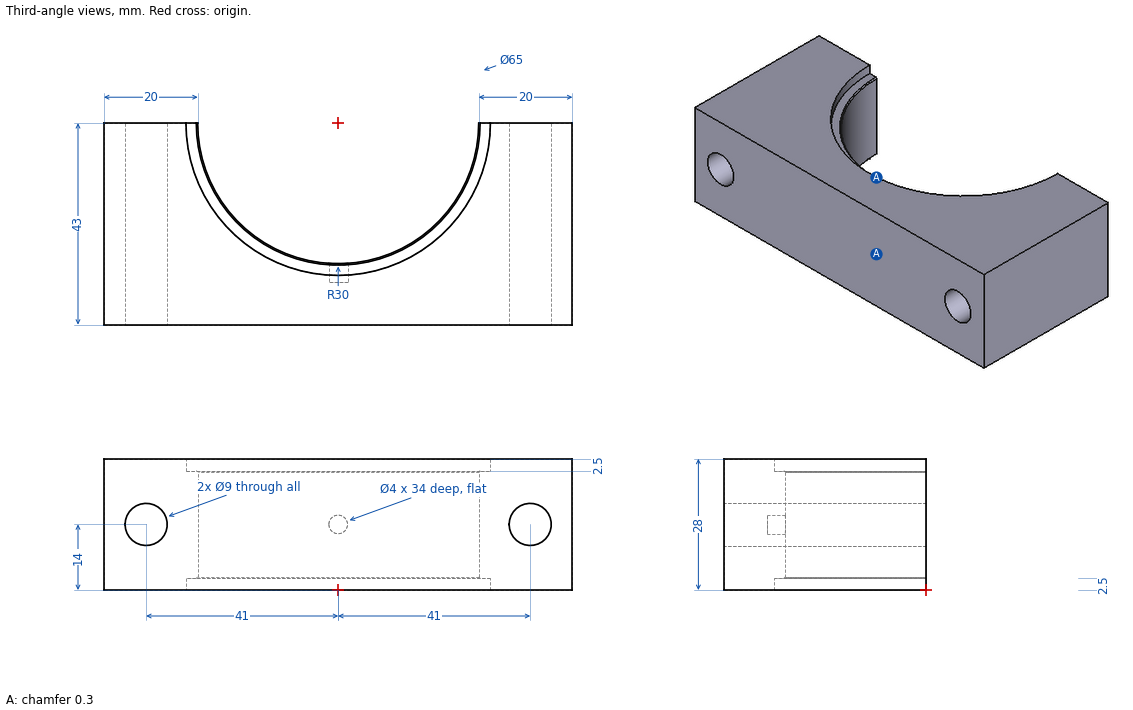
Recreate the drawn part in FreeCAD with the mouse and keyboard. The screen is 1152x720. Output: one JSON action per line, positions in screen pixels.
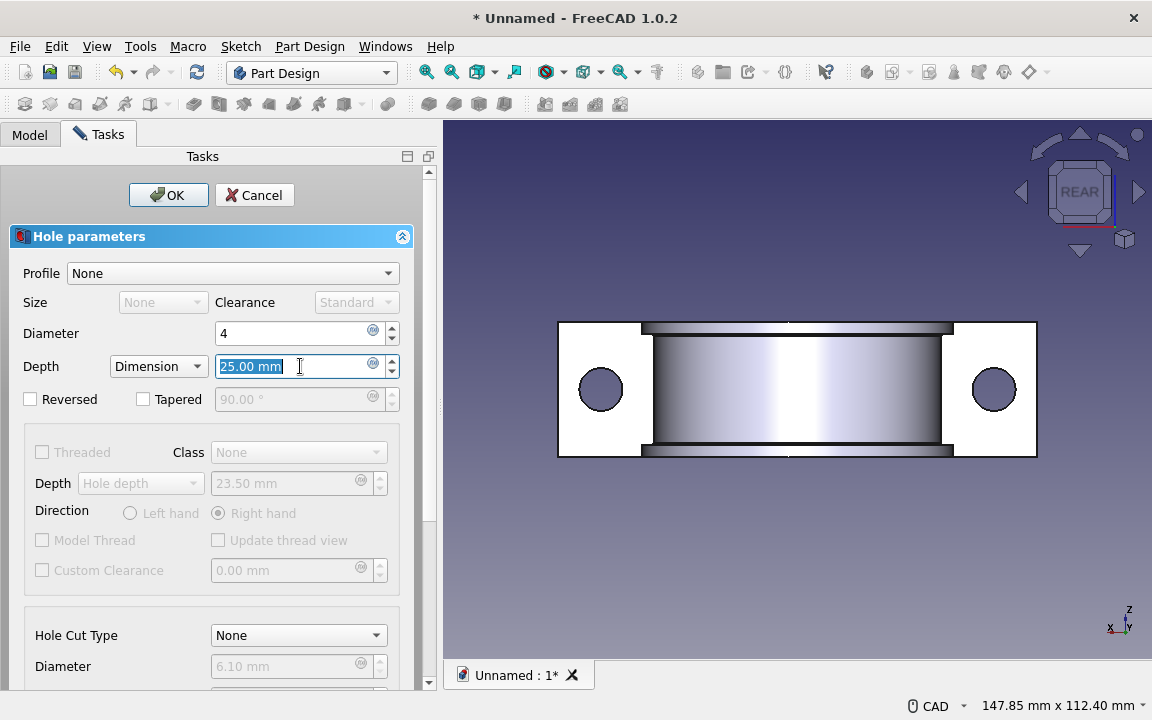
{"action": "type", "text": "34"}
{"action": "key", "text": "Tab"}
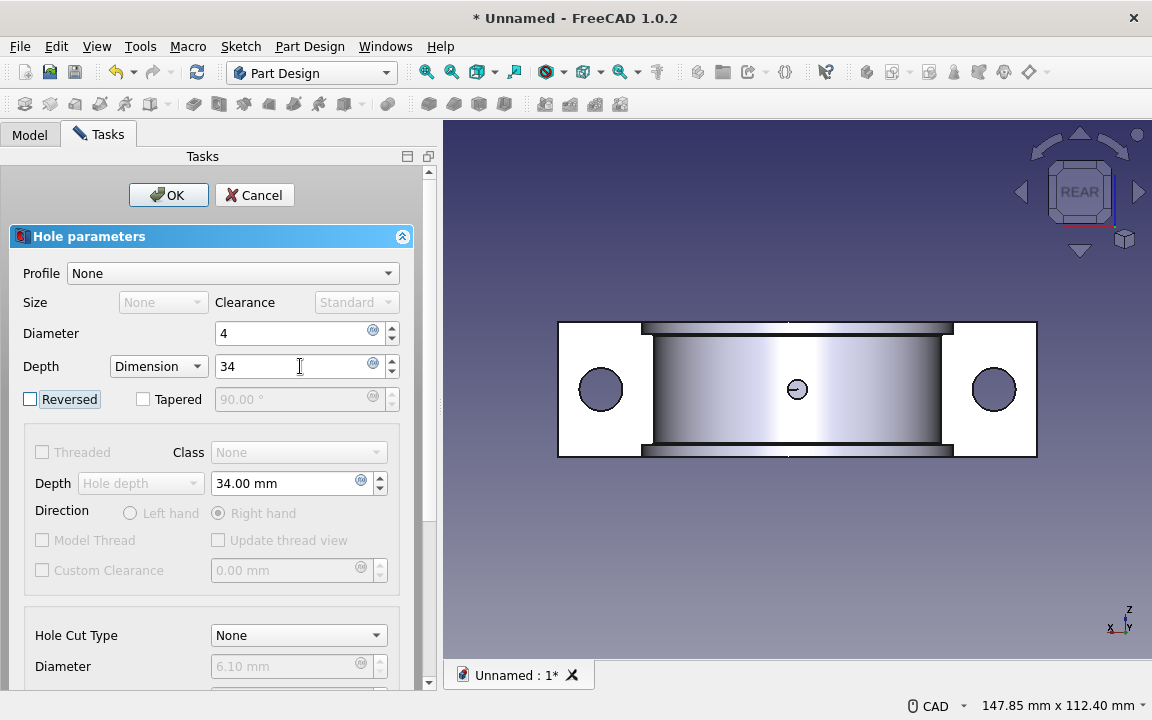
{"action": "scroll", "coordinate": [429, 428], "scroll_direction": "down", "scroll_amount": 4}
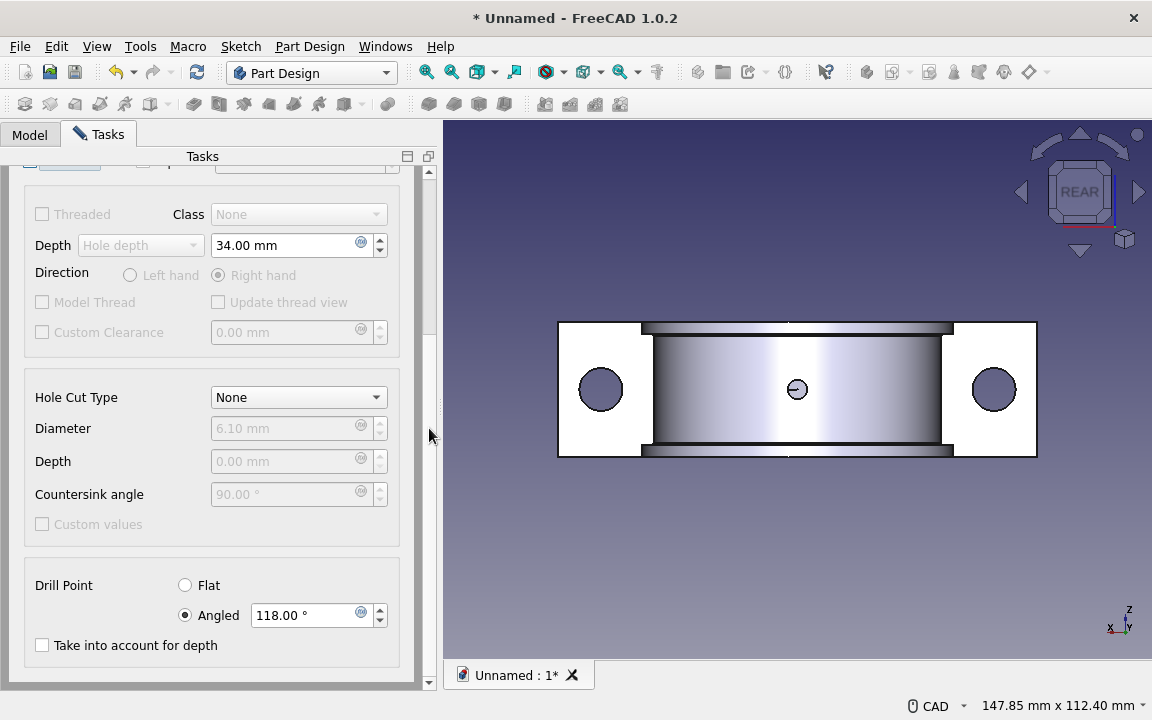
{"action": "left_click", "coordinate": [186, 583]}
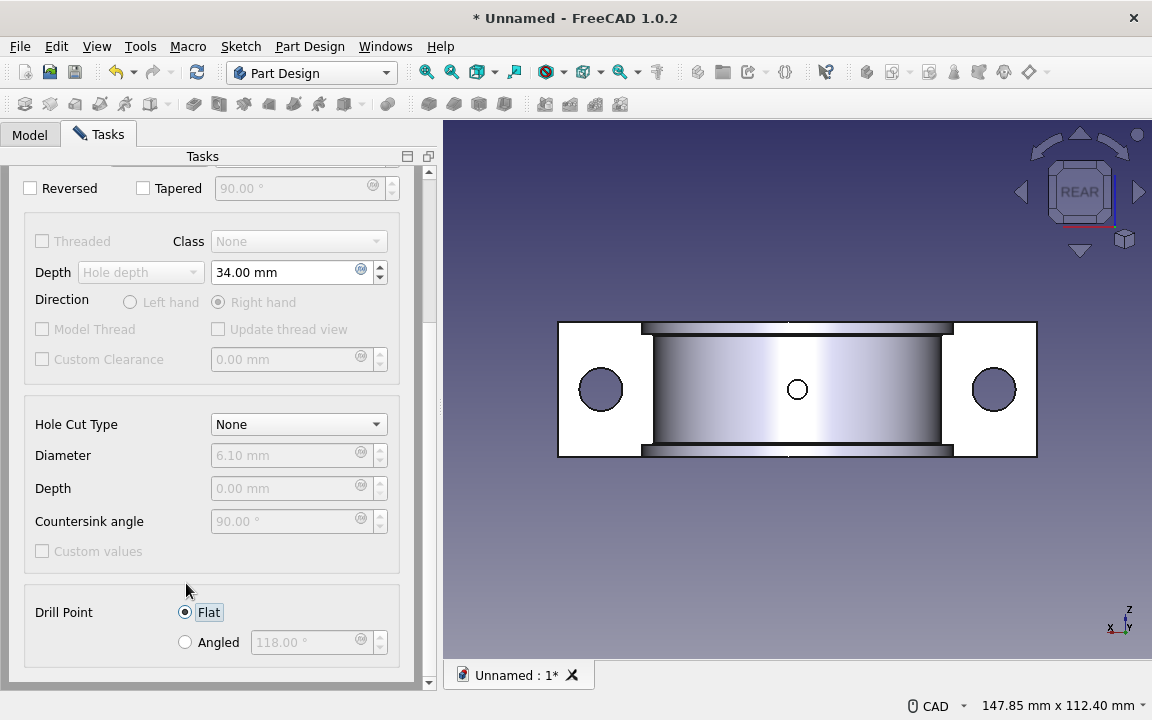
{"action": "scroll", "coordinate": [429, 428], "scroll_direction": "up", "scroll_amount": 5}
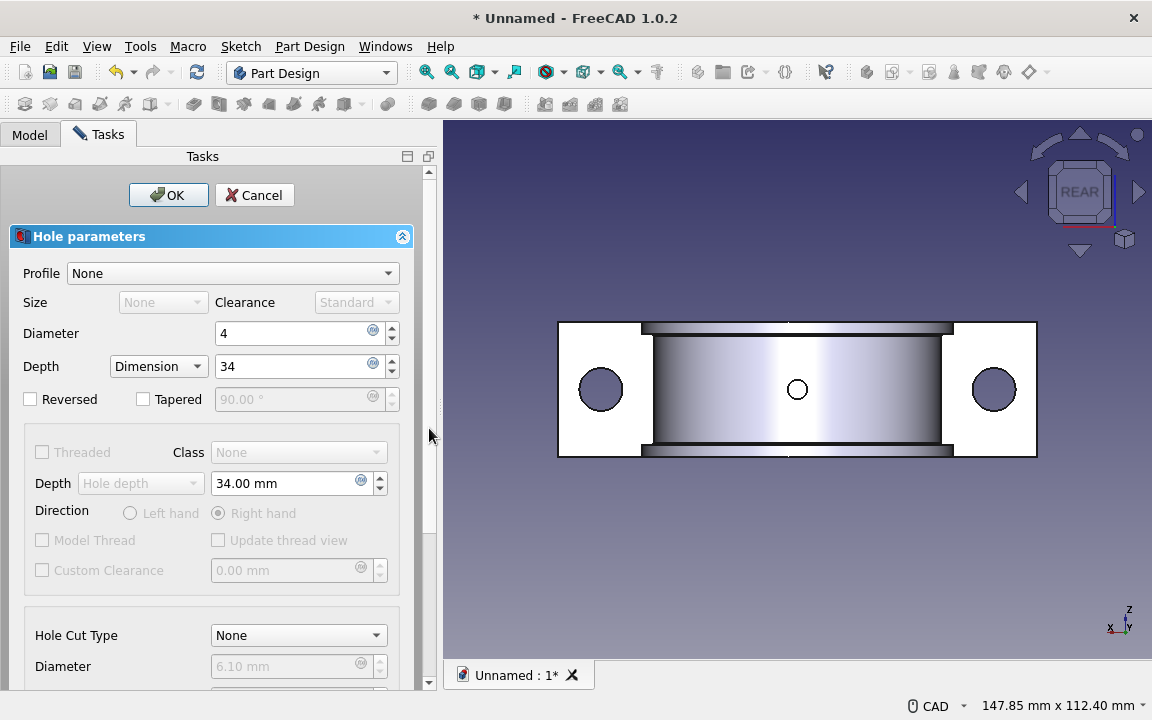
{"action": "left_click", "coordinate": [169, 195]}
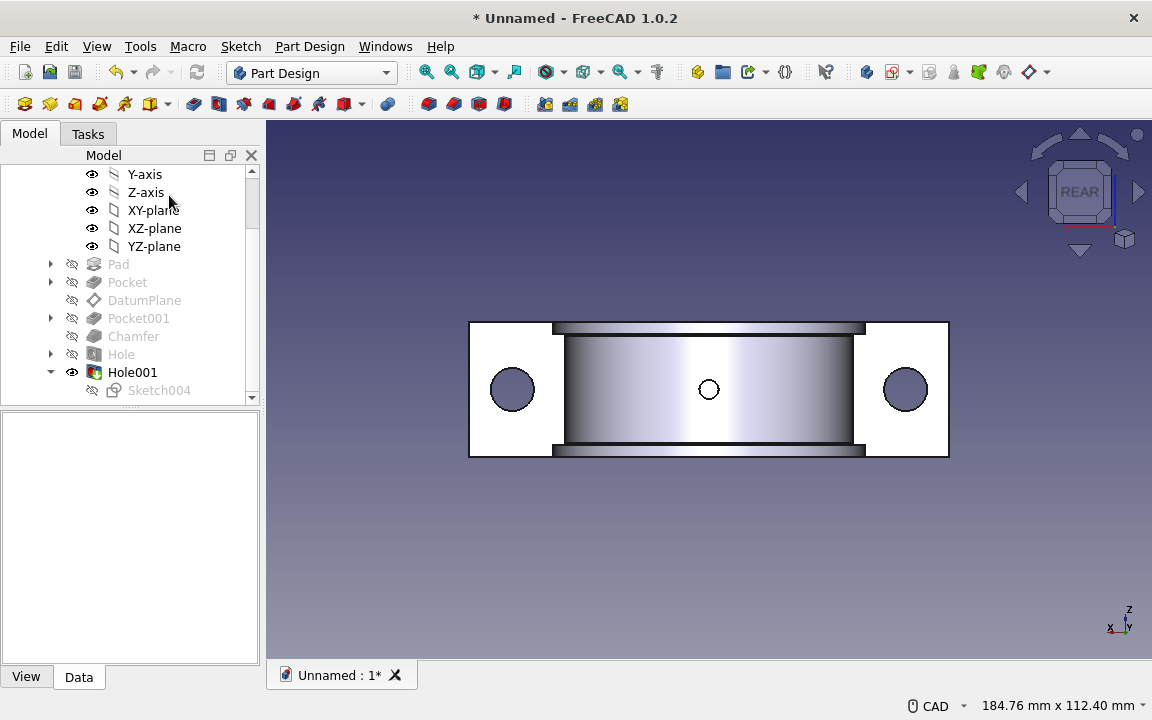
{"action": "key", "text": "0"}